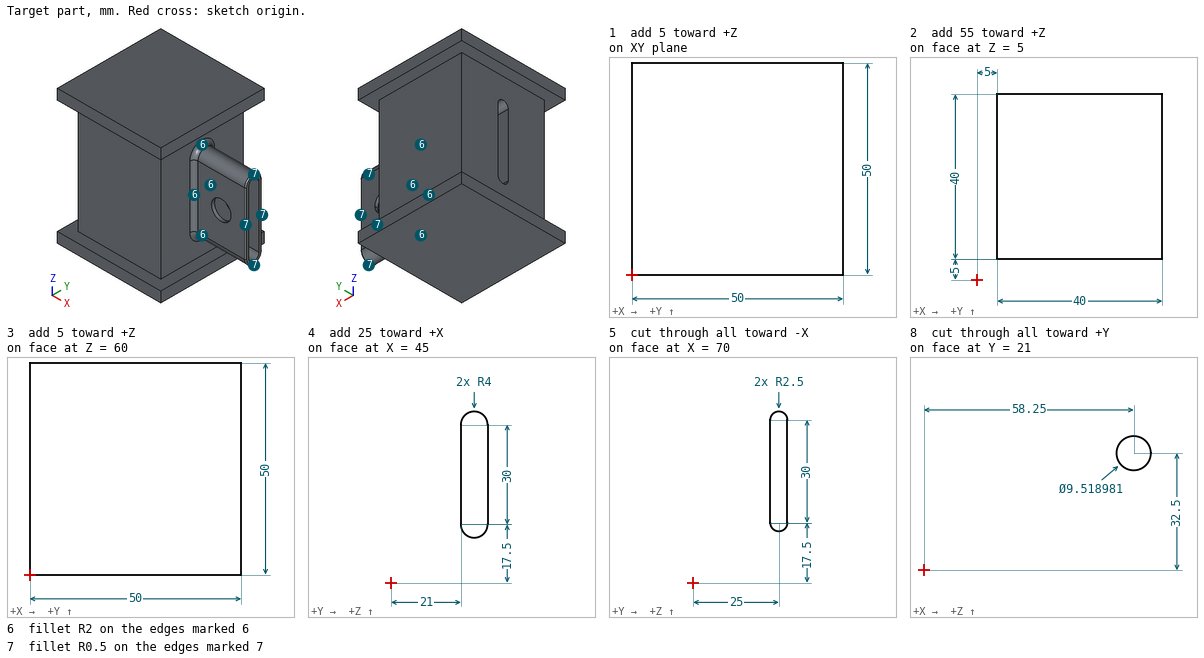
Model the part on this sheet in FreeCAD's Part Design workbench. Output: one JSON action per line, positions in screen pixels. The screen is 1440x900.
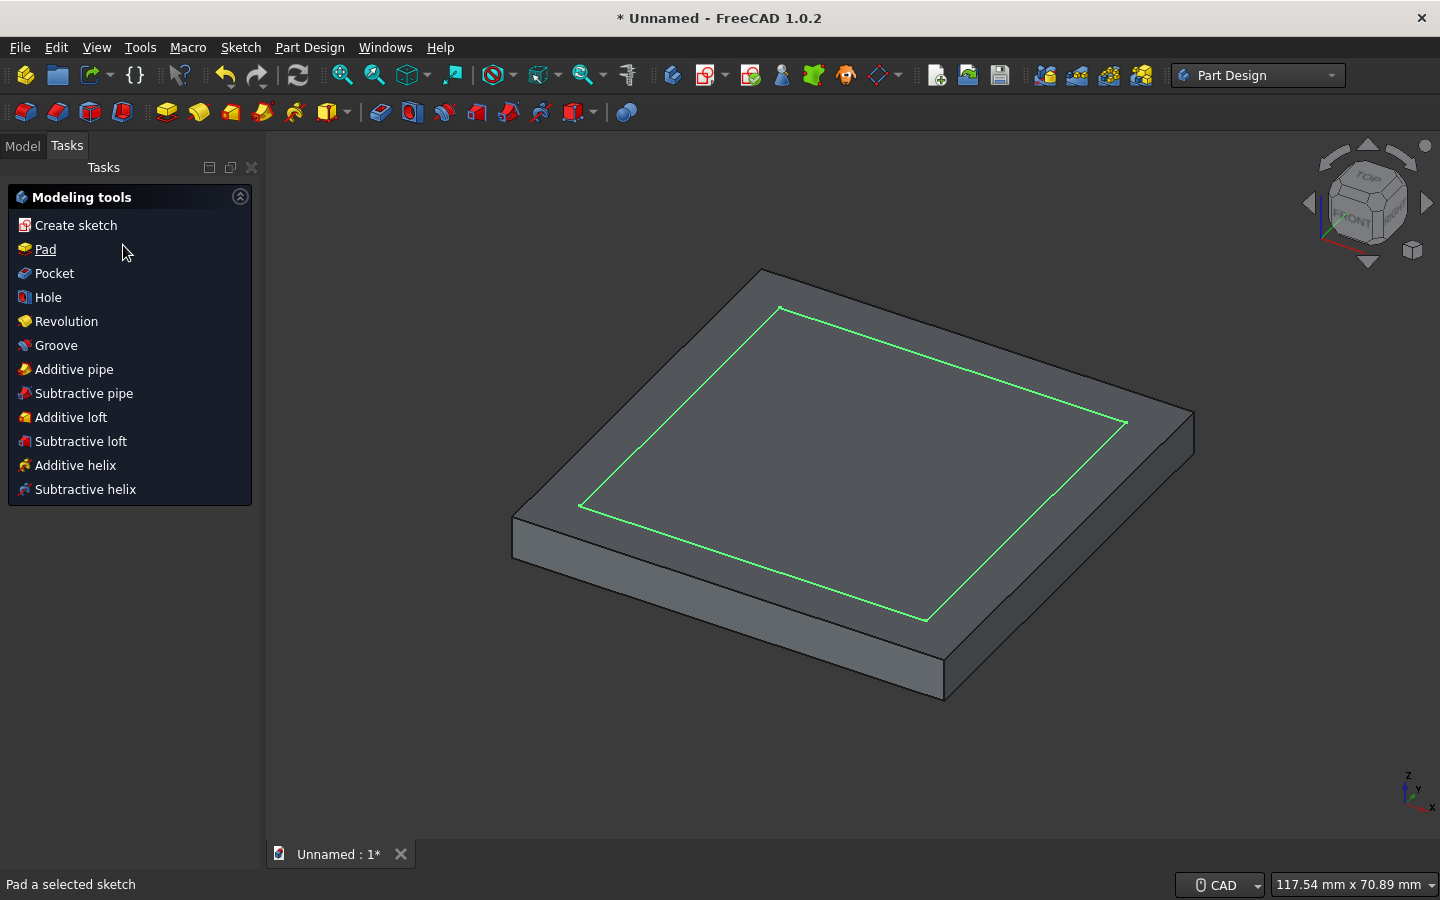
{"action": "left_click", "coordinate": [168, 112]}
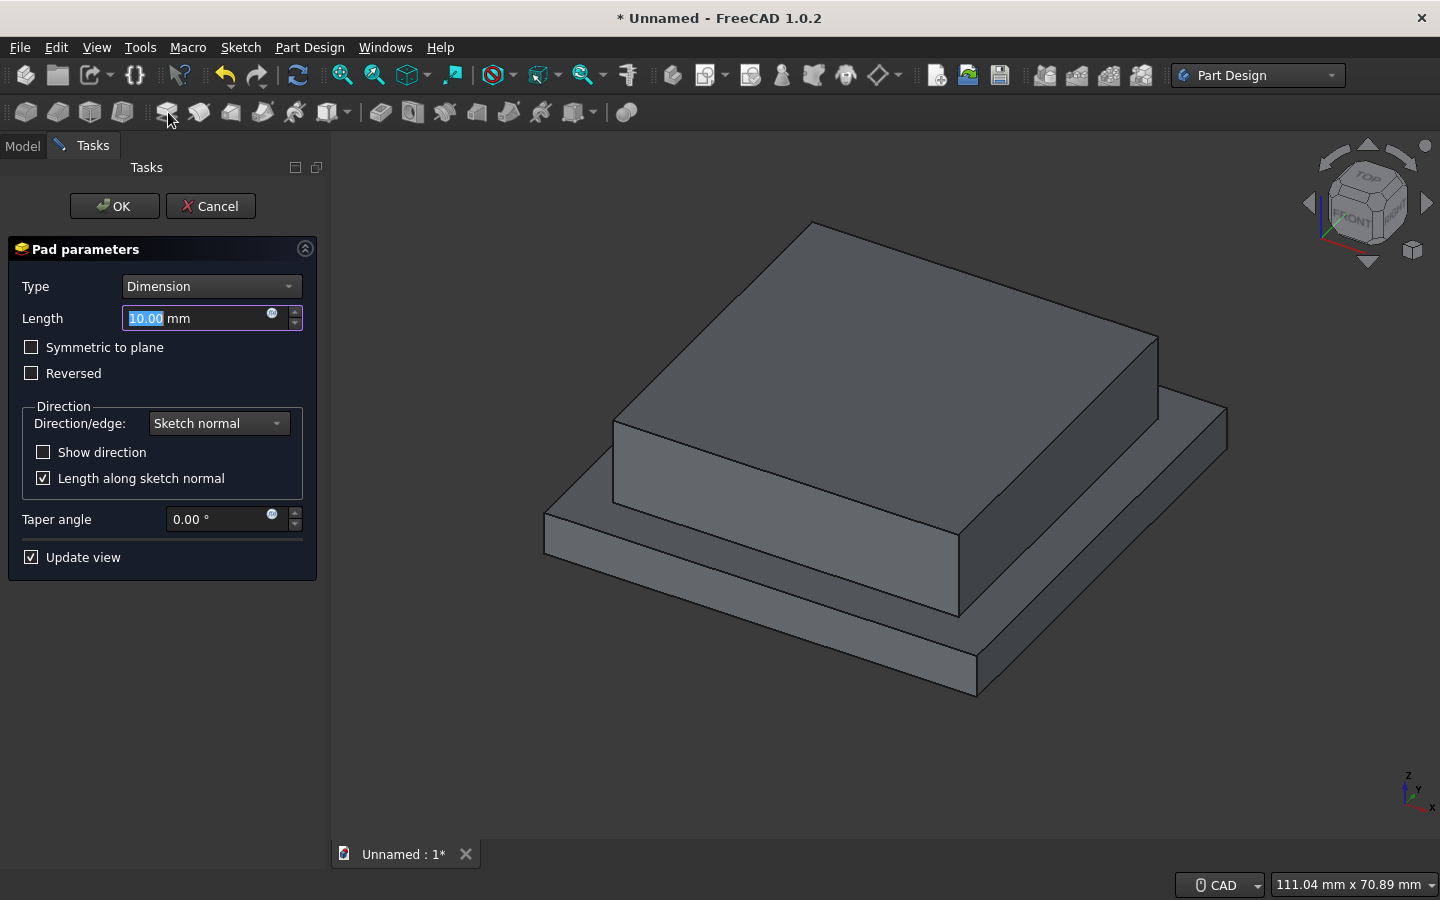
{"action": "type", "text": "55"}
{"action": "key", "text": "Tab"}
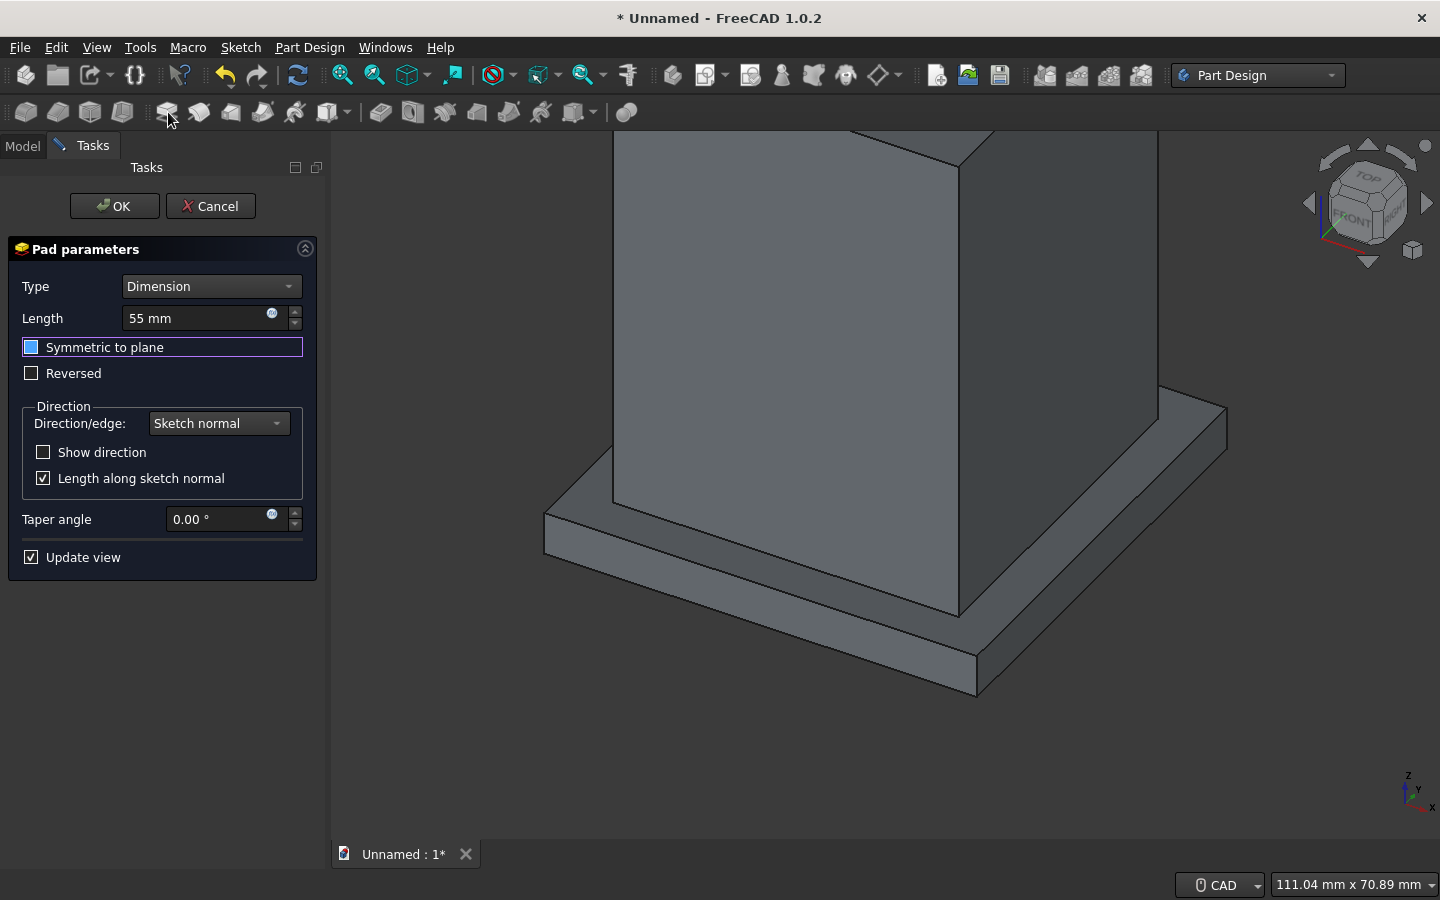
{"action": "left_click", "coordinate": [115, 206]}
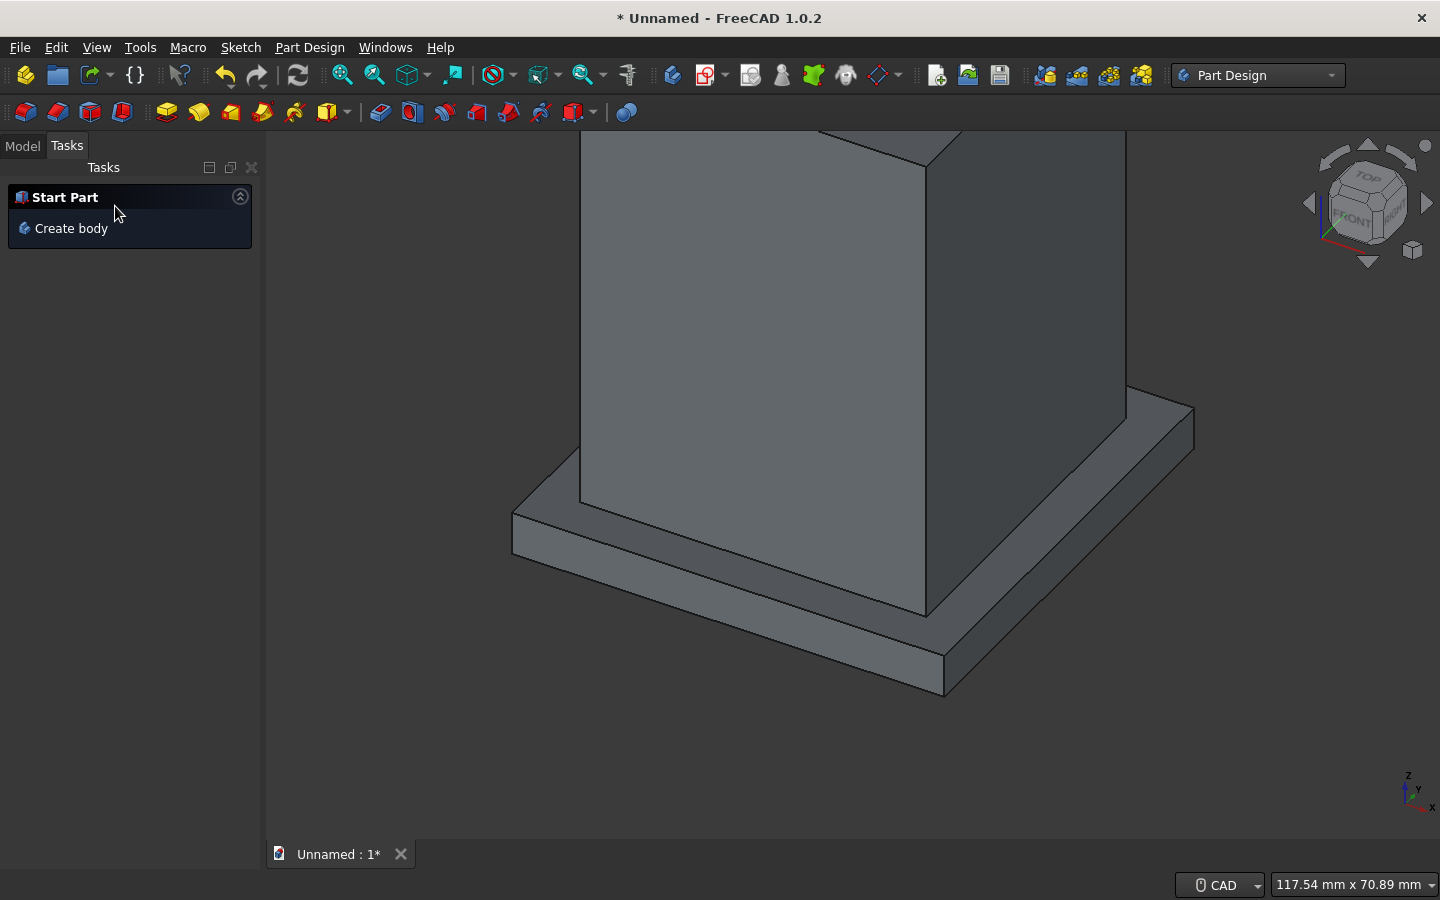
{"action": "left_click", "coordinate": [344, 76]}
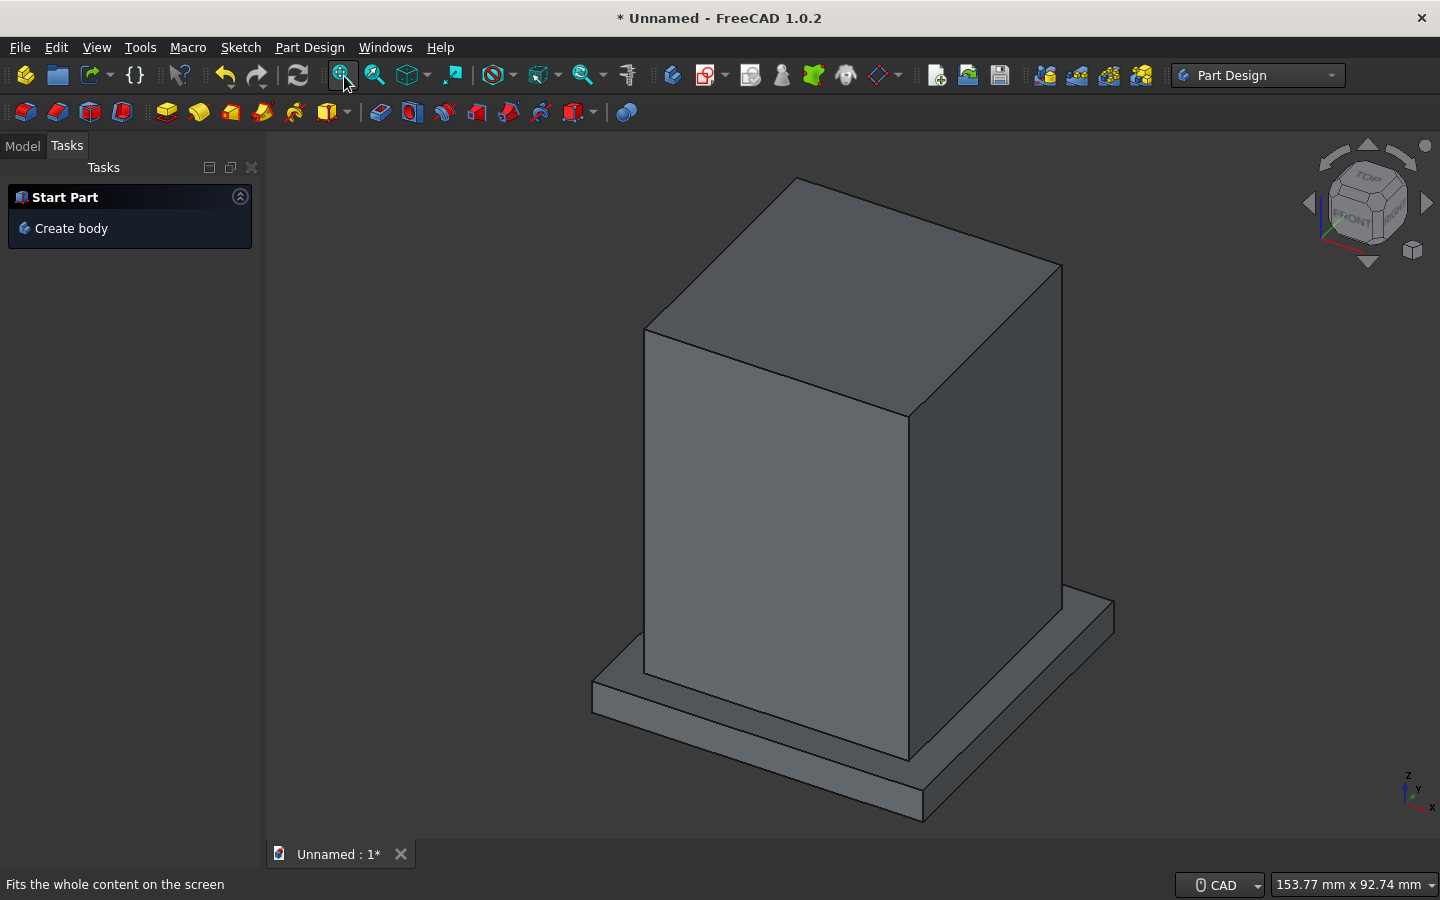
{"action": "left_click", "coordinate": [853, 296]}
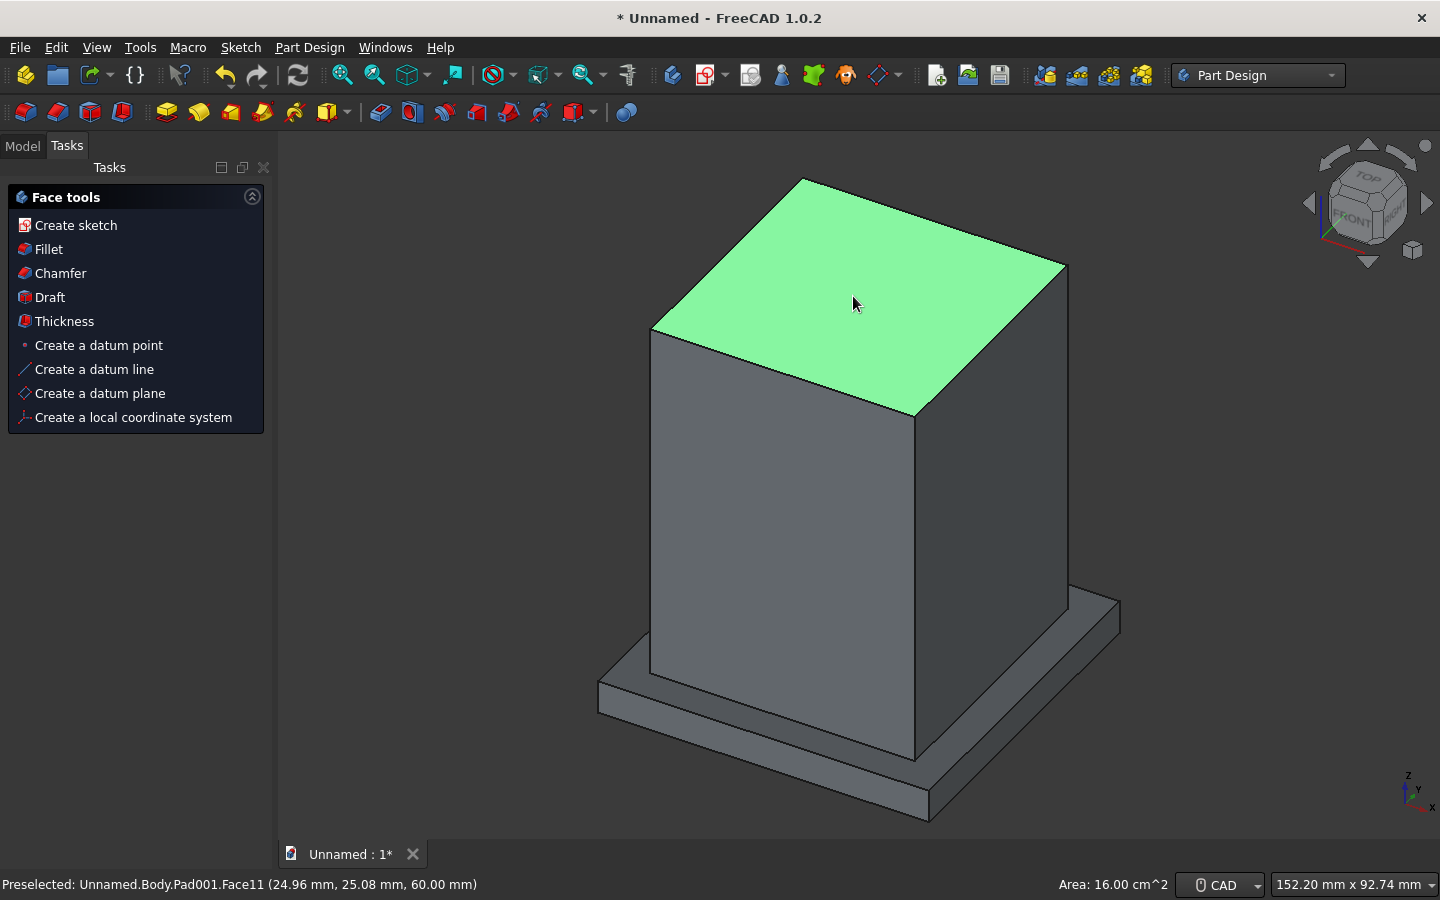
{"action": "left_click", "coordinate": [706, 76]}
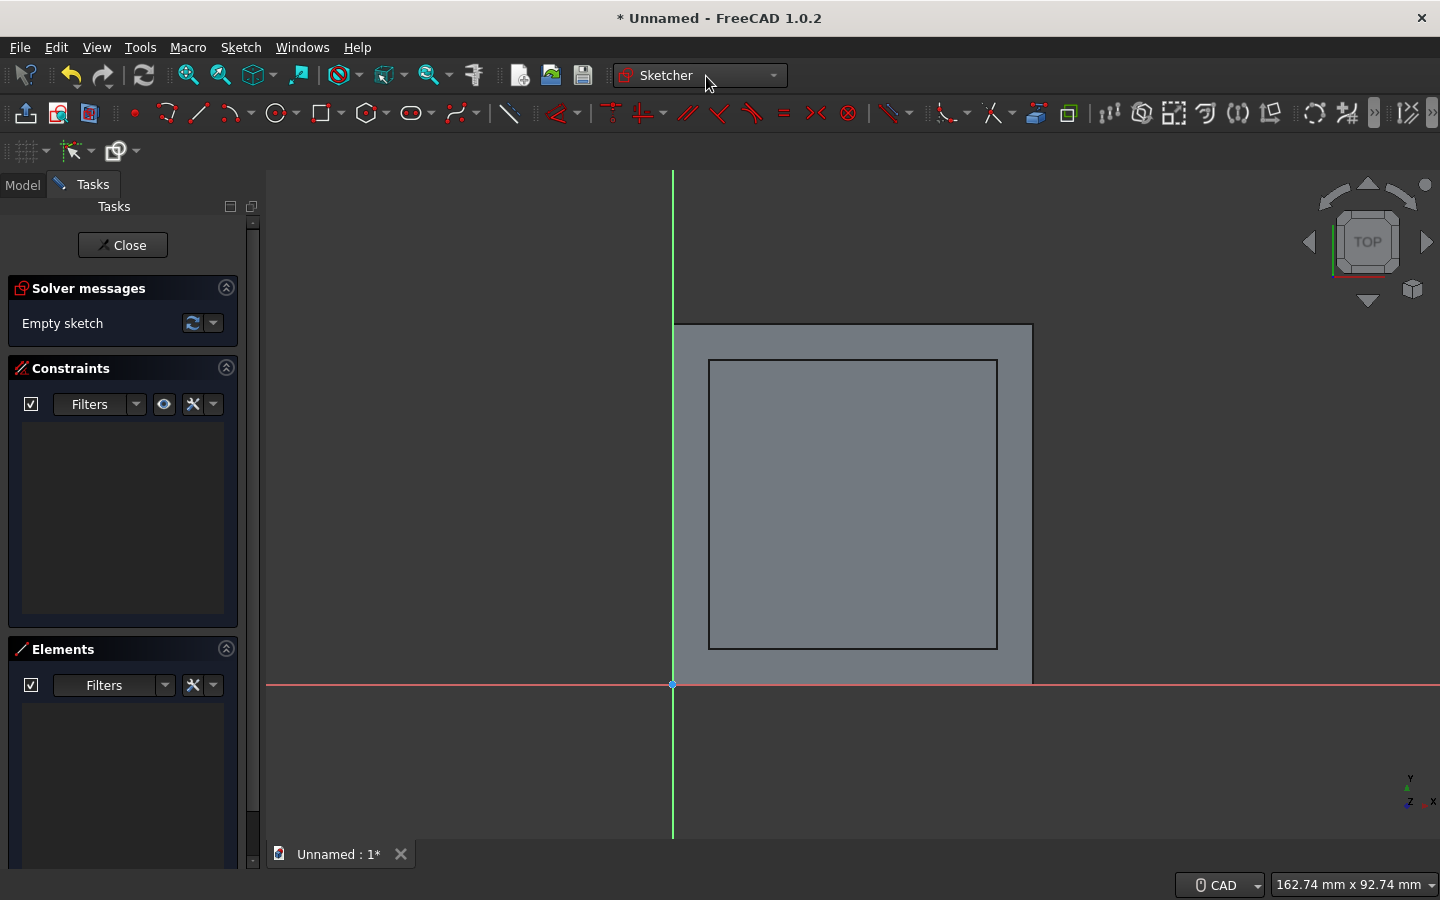
{"action": "left_click", "coordinate": [322, 114]}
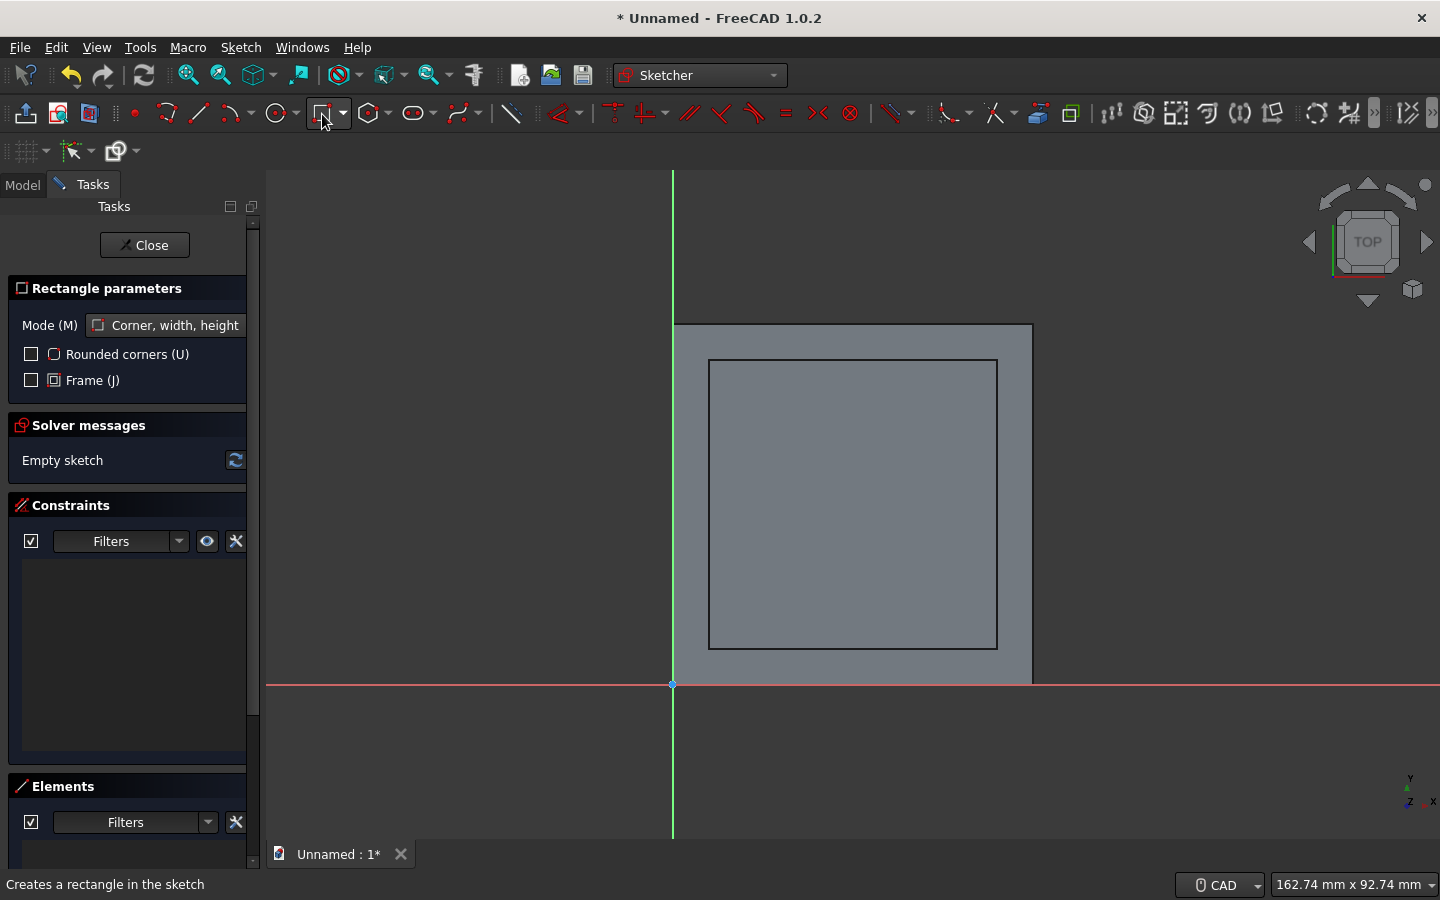
{"action": "left_click", "coordinate": [673, 685]}
{"action": "left_click", "coordinate": [1033, 324]}
{"action": "key", "text": "Escape"}